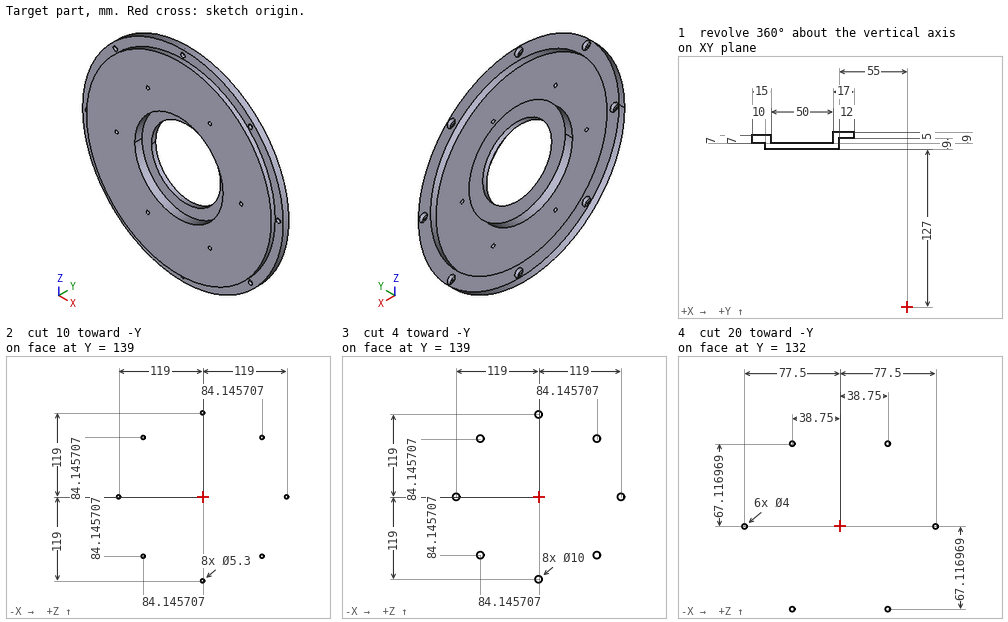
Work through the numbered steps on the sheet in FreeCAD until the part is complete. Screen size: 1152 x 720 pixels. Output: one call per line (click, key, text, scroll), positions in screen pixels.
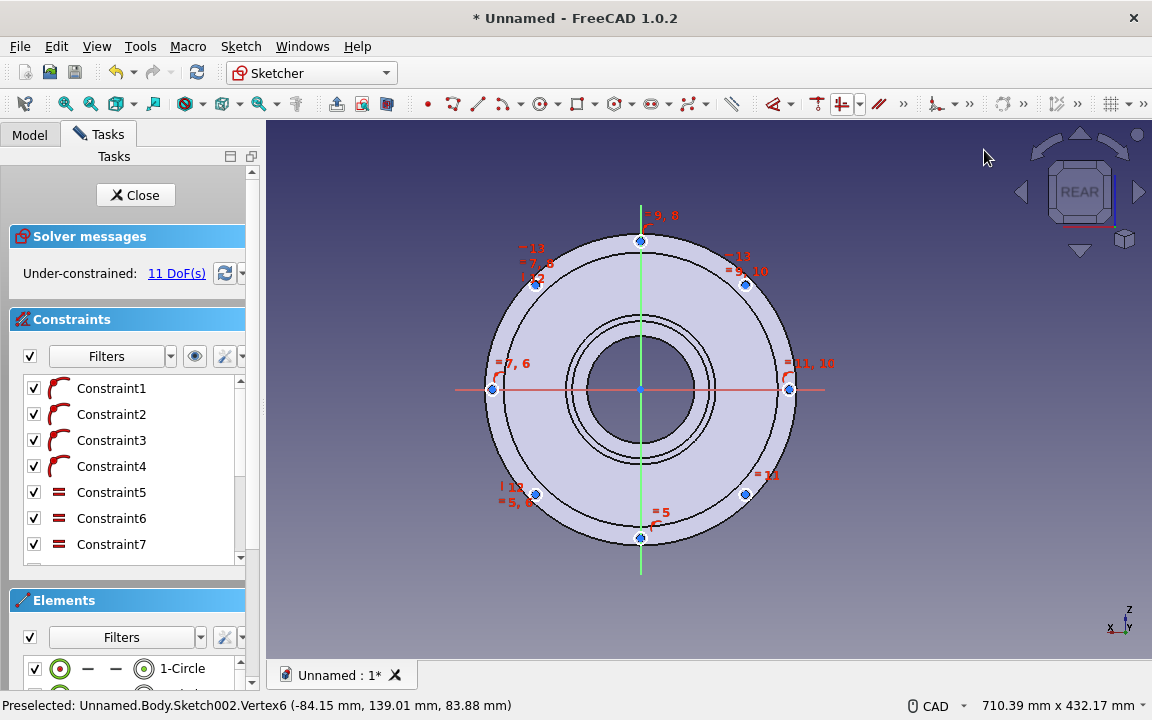
click(746, 285)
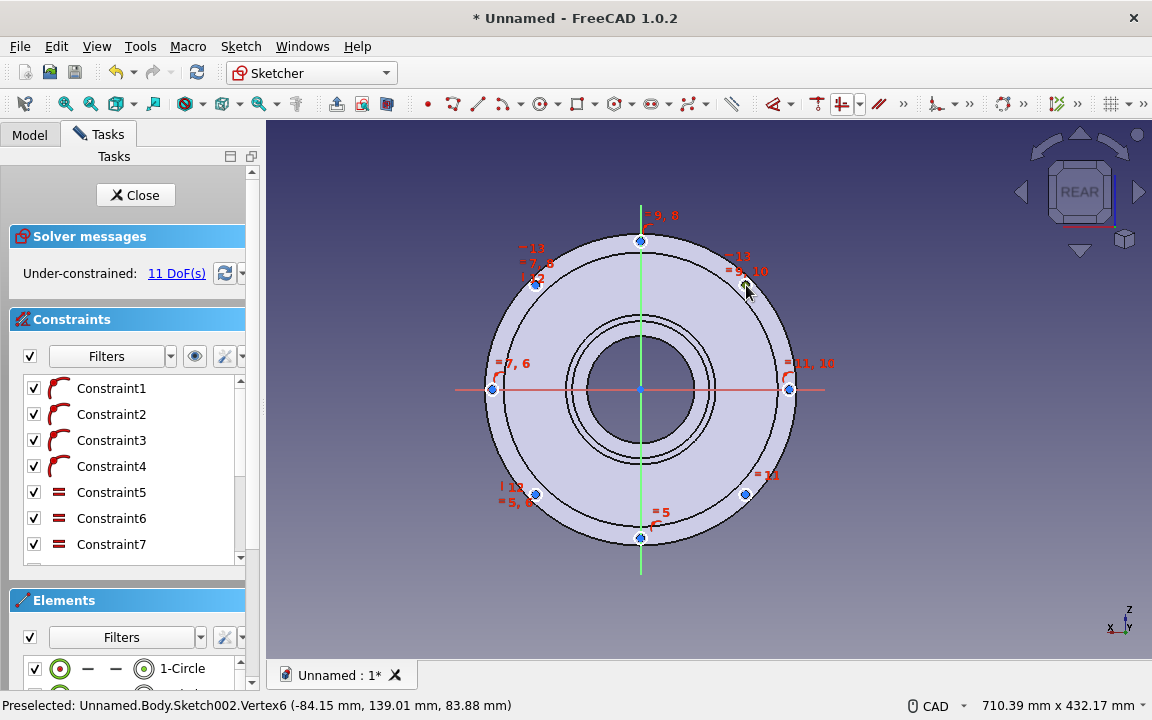
click(746, 495)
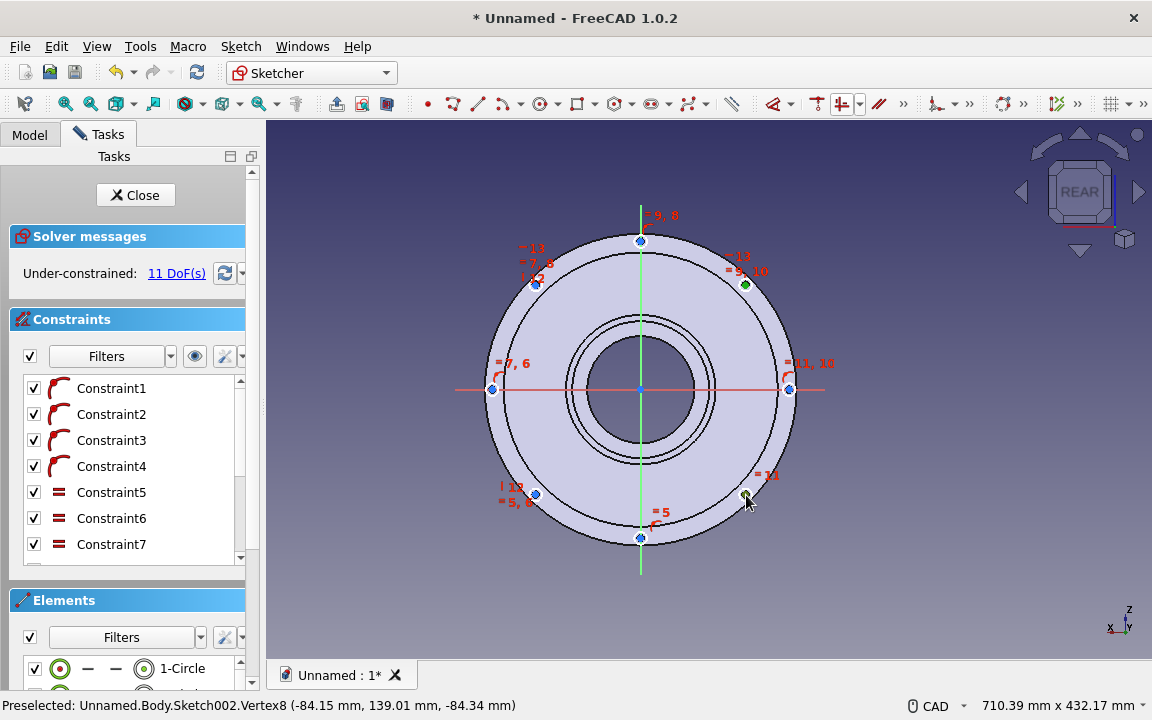
click(860, 104)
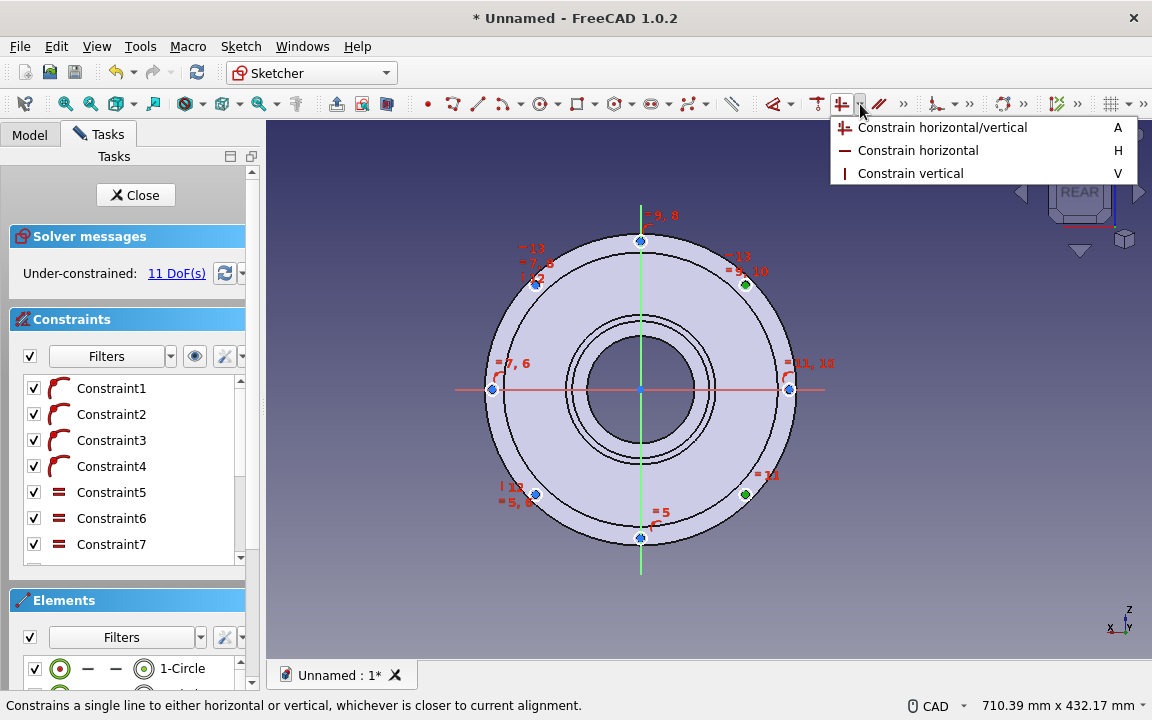
click(984, 174)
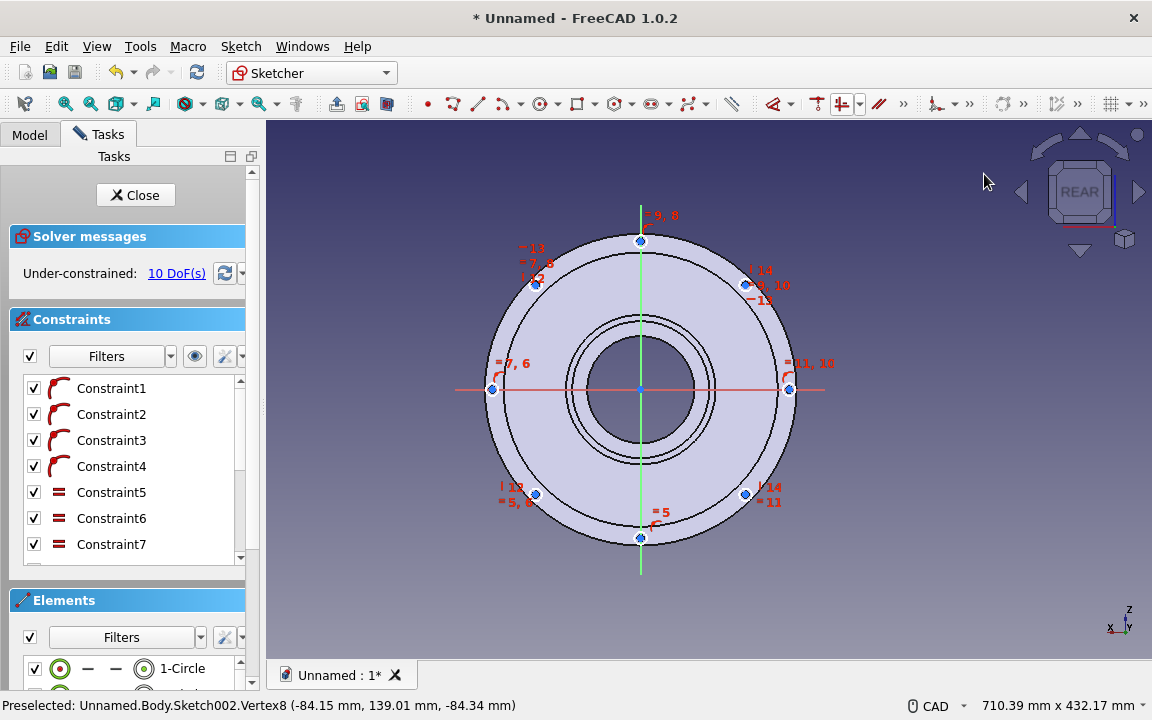
click(536, 495)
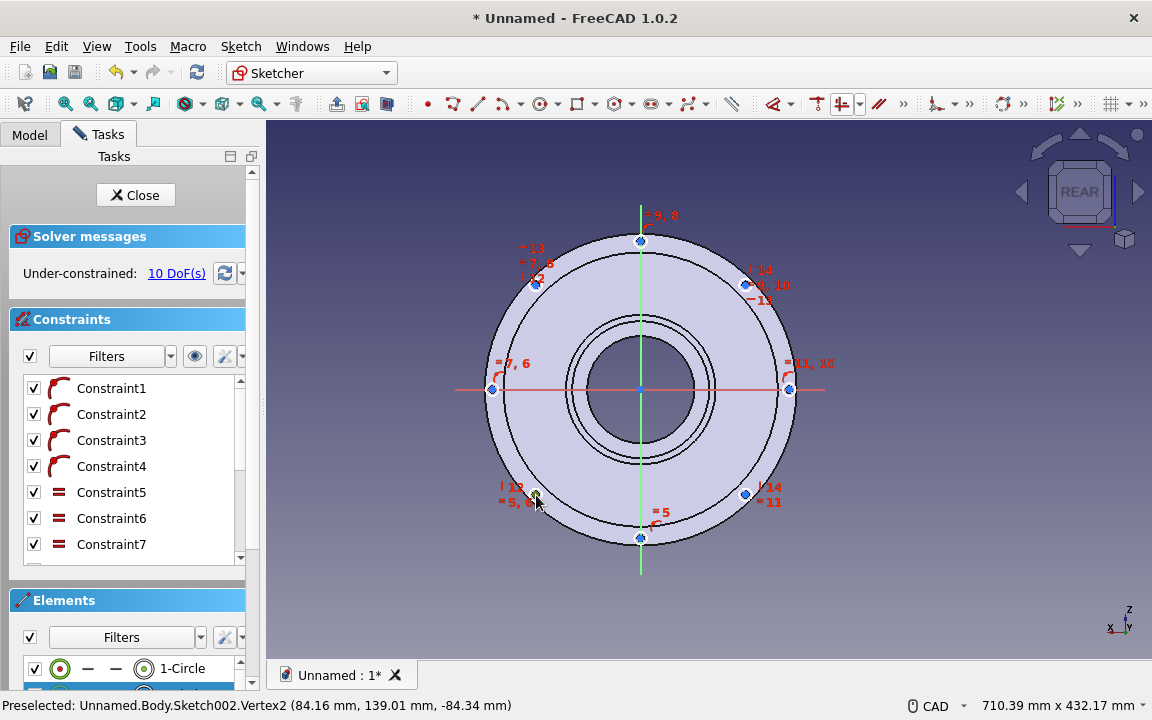
click(746, 495)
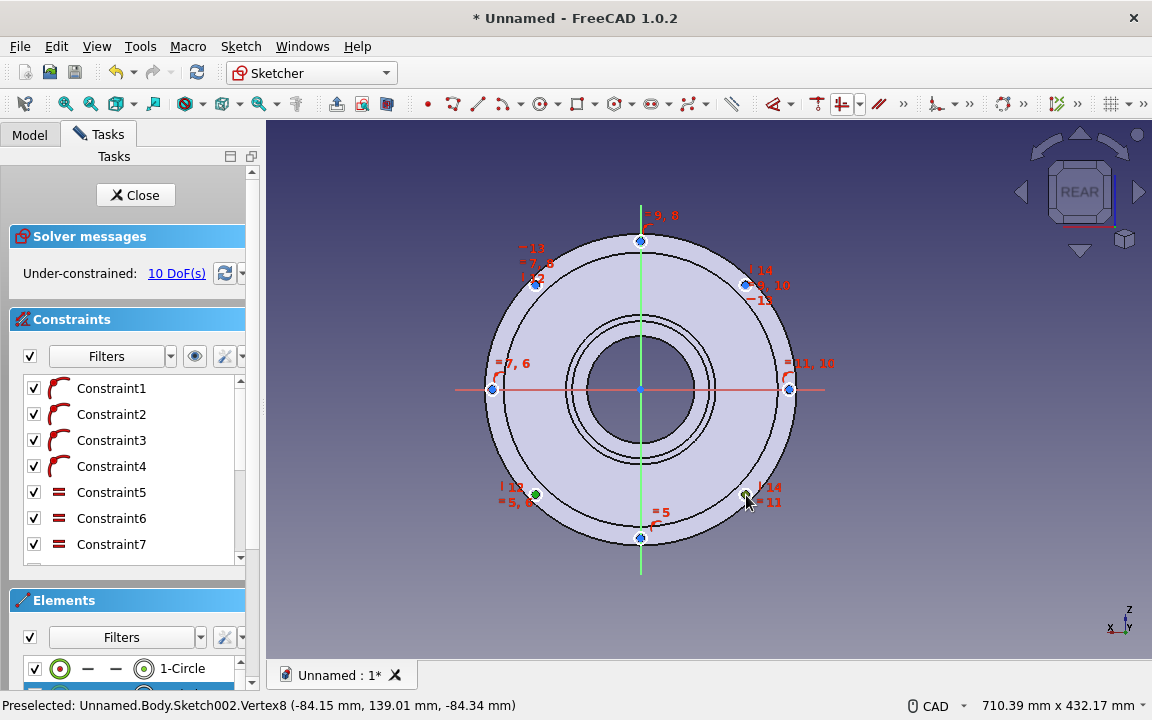
click(860, 104)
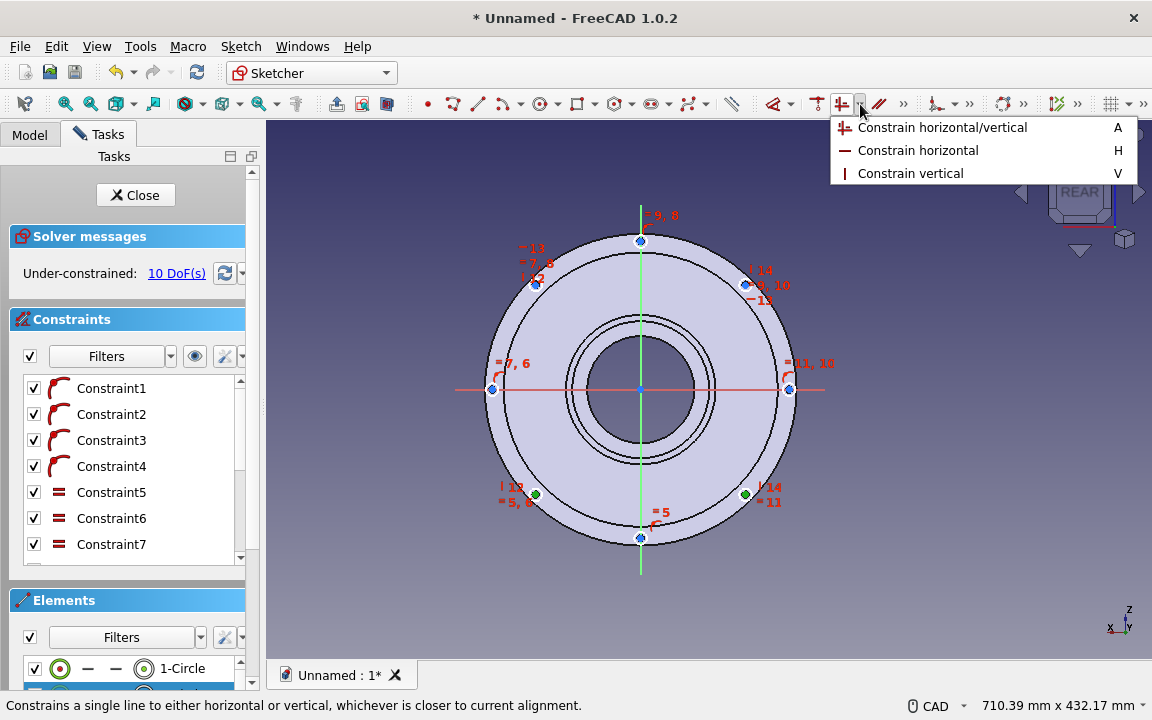
click(984, 150)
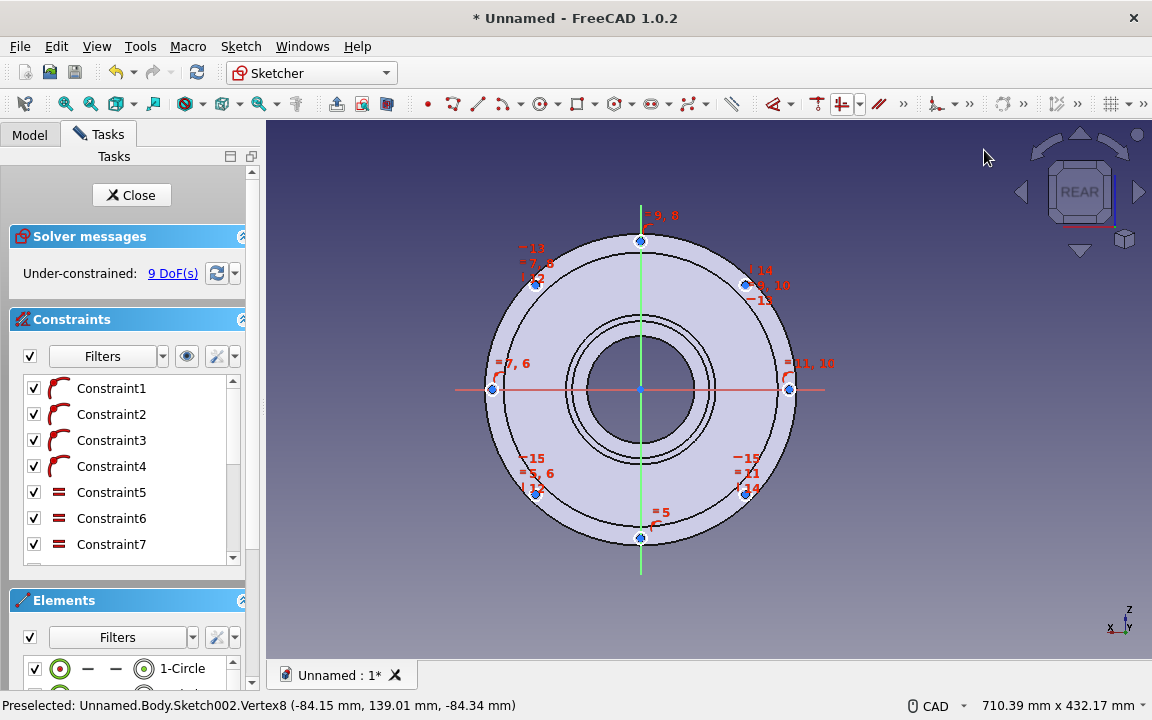
click(772, 104)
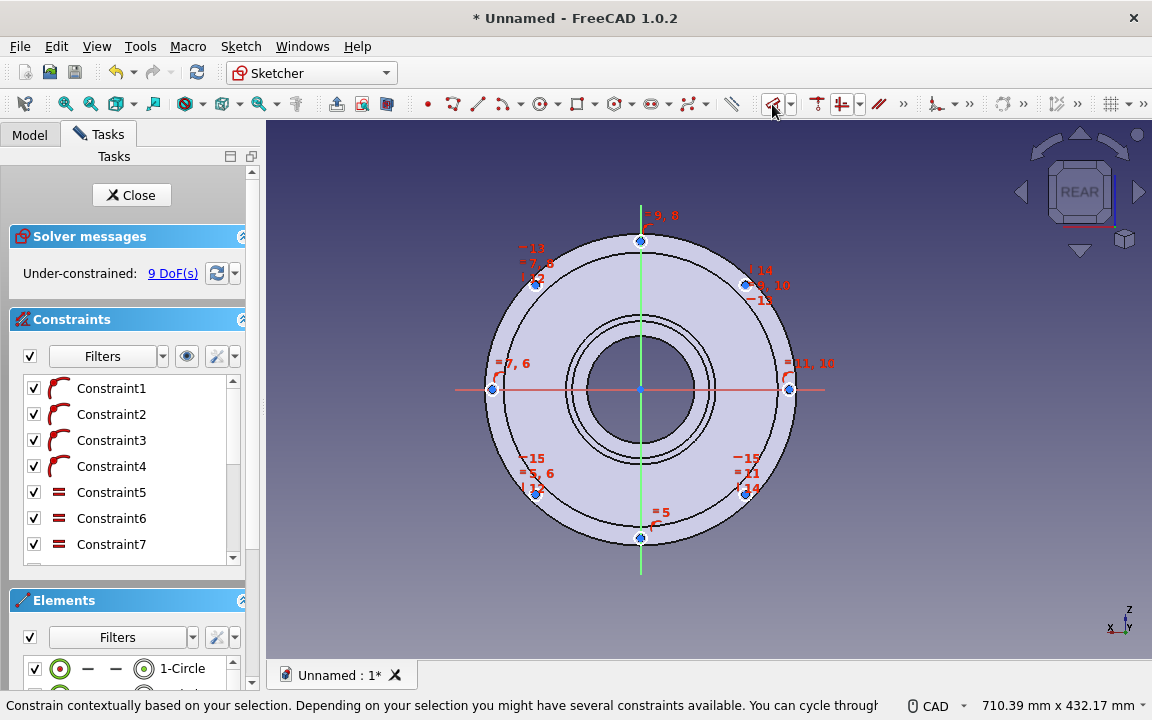
scroll(641, 532, up, 6)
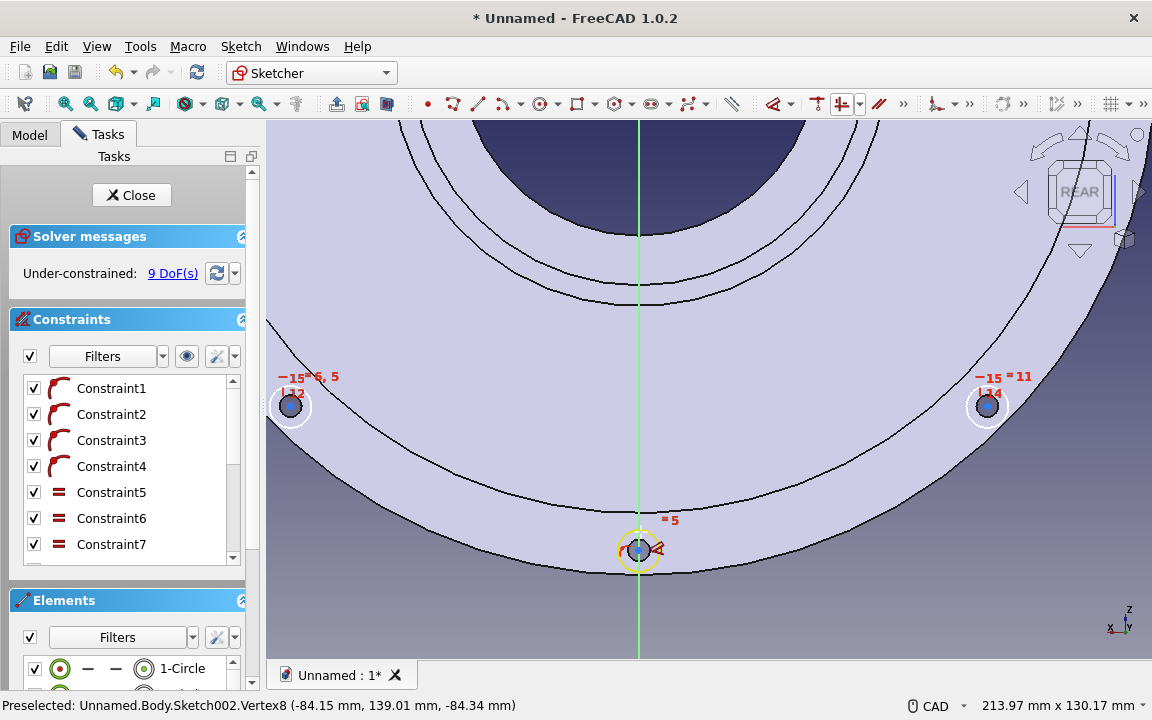
click(640, 530)
click(667, 506)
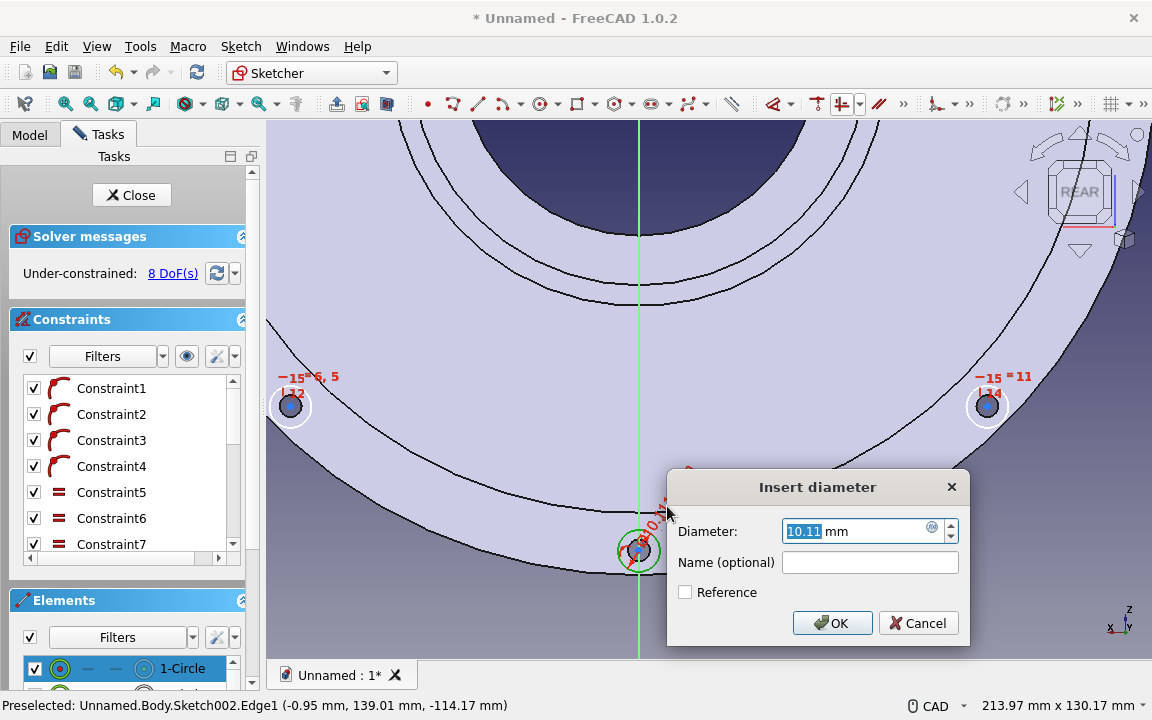
text(10)
key(Return)